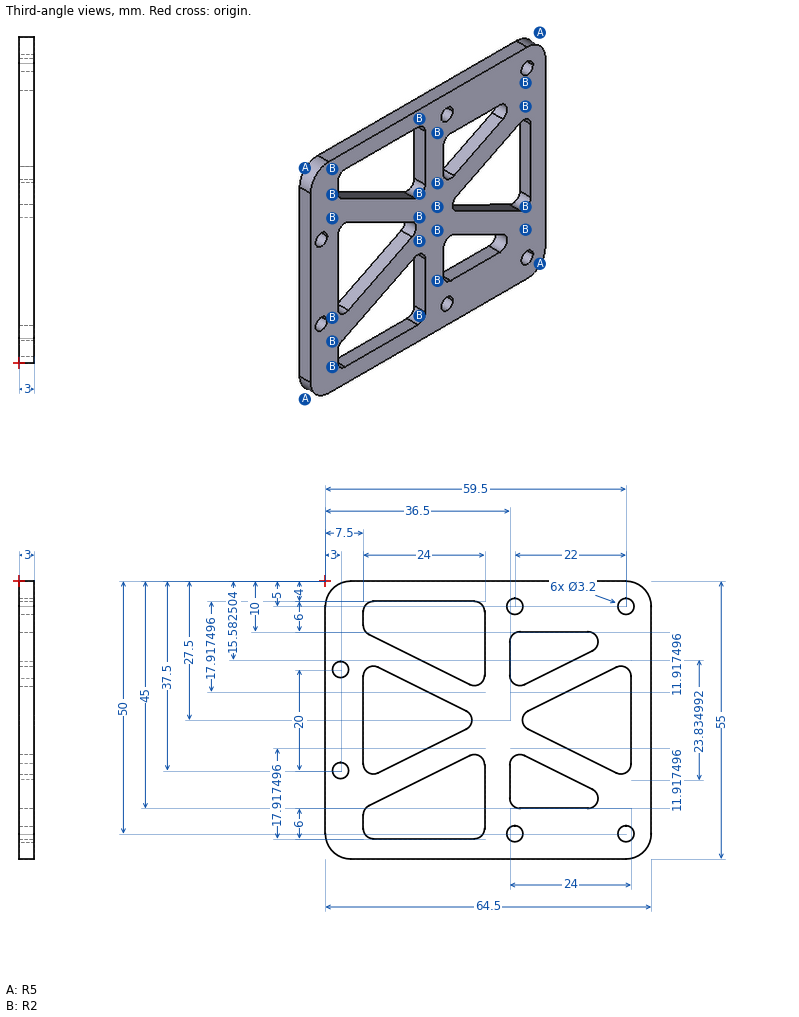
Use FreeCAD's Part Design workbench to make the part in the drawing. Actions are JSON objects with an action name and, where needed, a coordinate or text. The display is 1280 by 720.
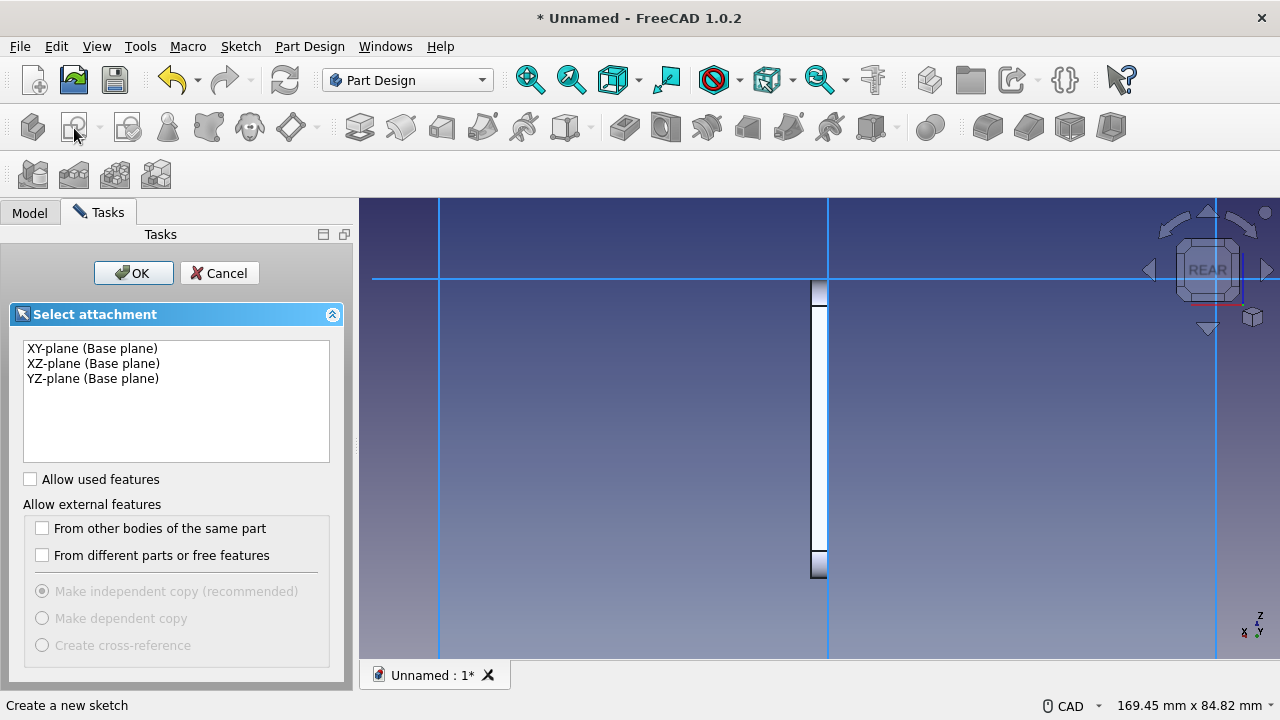
{"action": "left_click", "coordinate": [84, 378]}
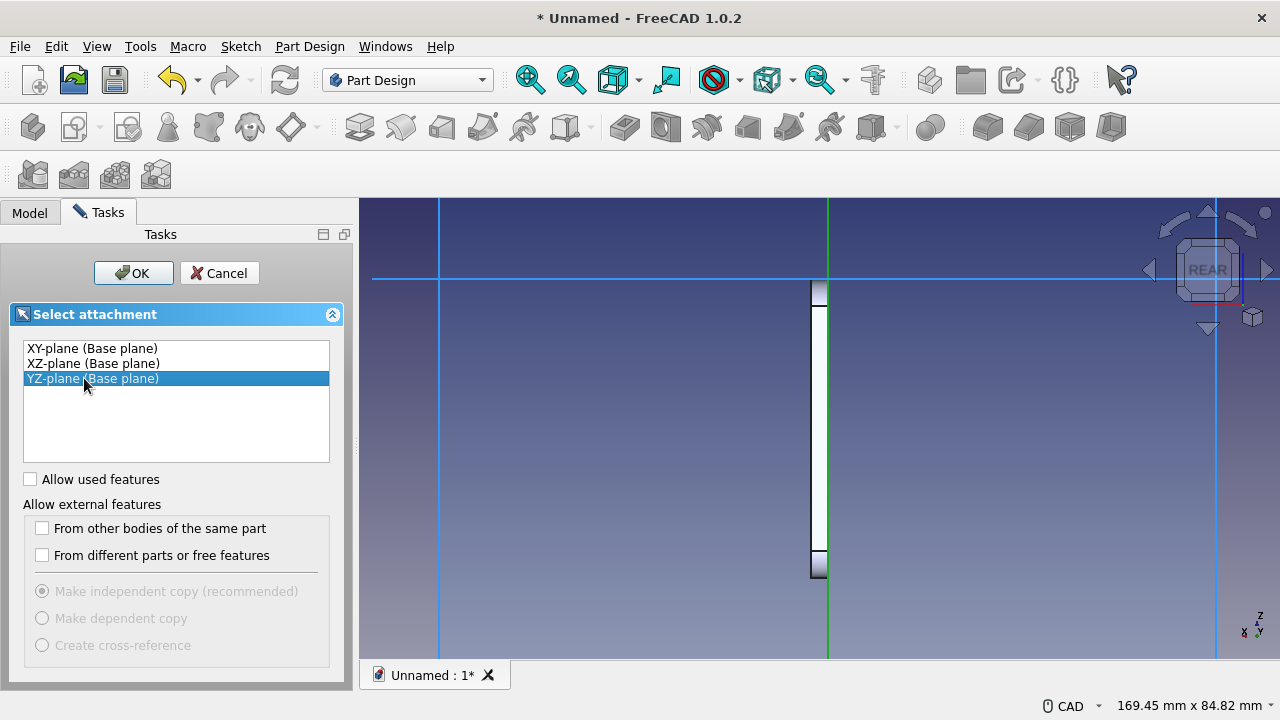
{"action": "left_click", "coordinate": [134, 273]}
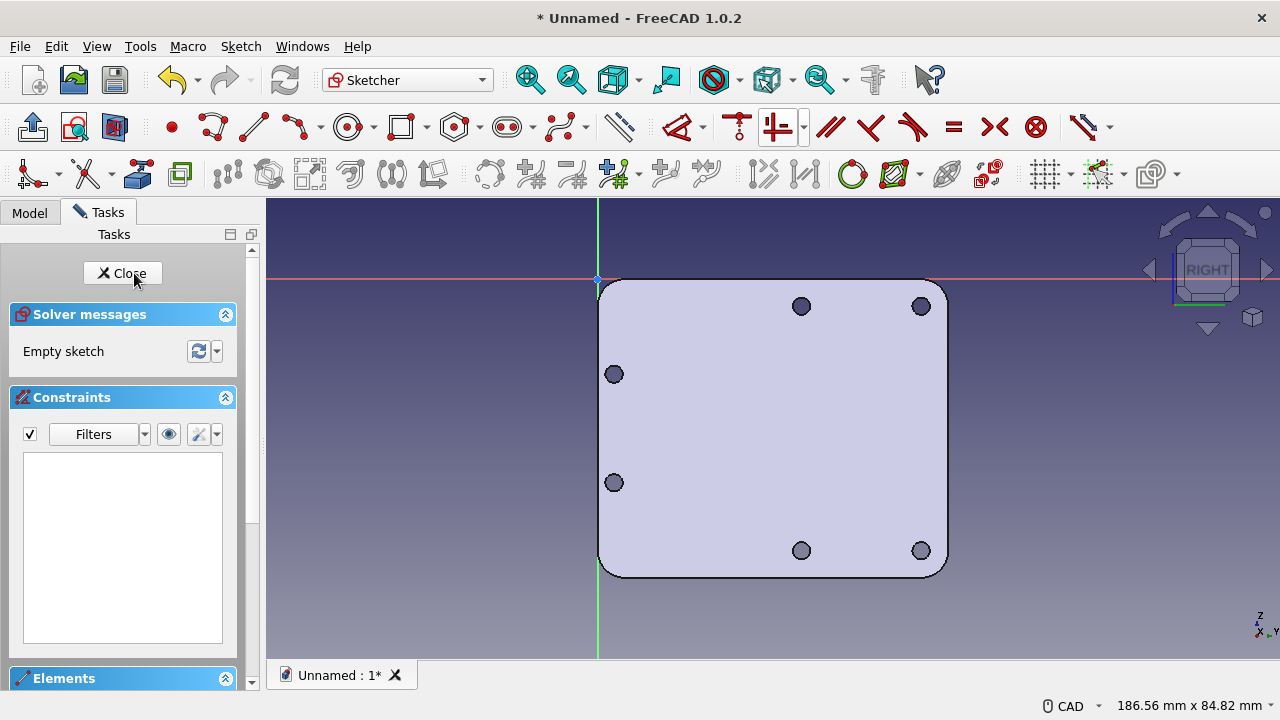
{"action": "key", "text": "q s"}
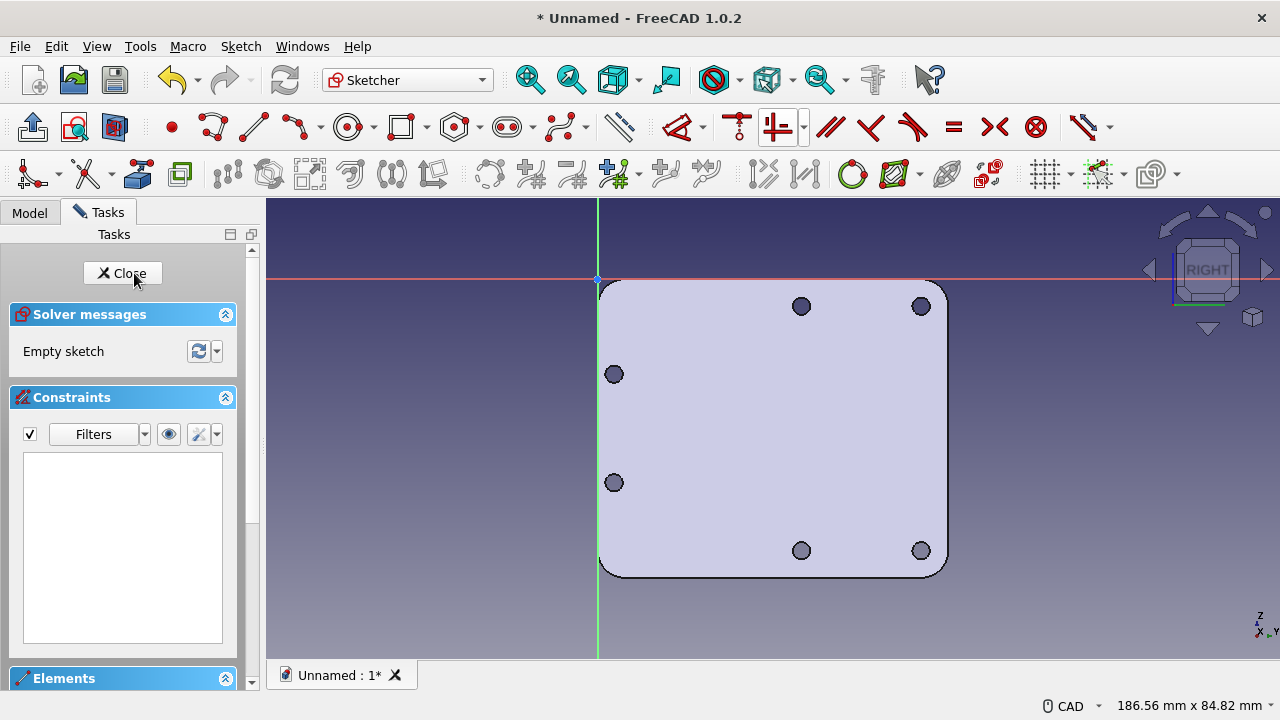
{"action": "key", "text": "g m"}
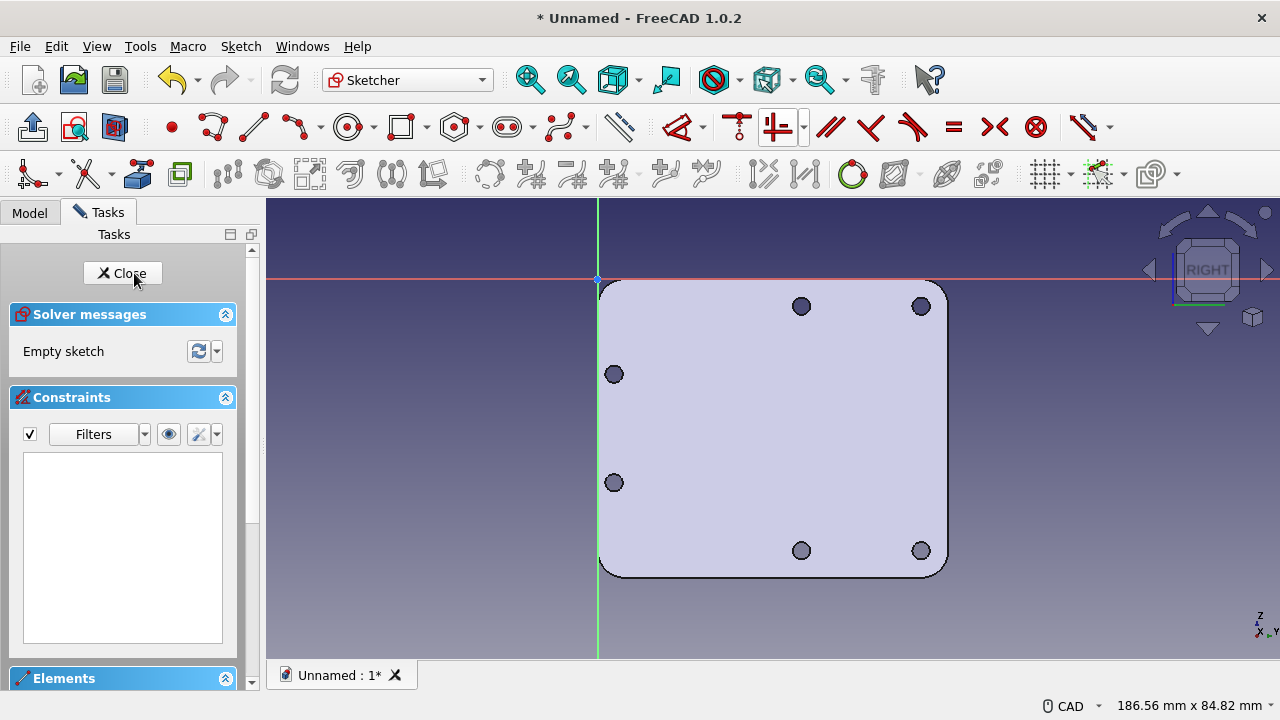
{"action": "left_click", "coordinate": [796, 428]}
{"action": "left_click", "coordinate": [927, 364]}
{"action": "left_click", "coordinate": [927, 493]}
{"action": "left_click", "coordinate": [796, 429]}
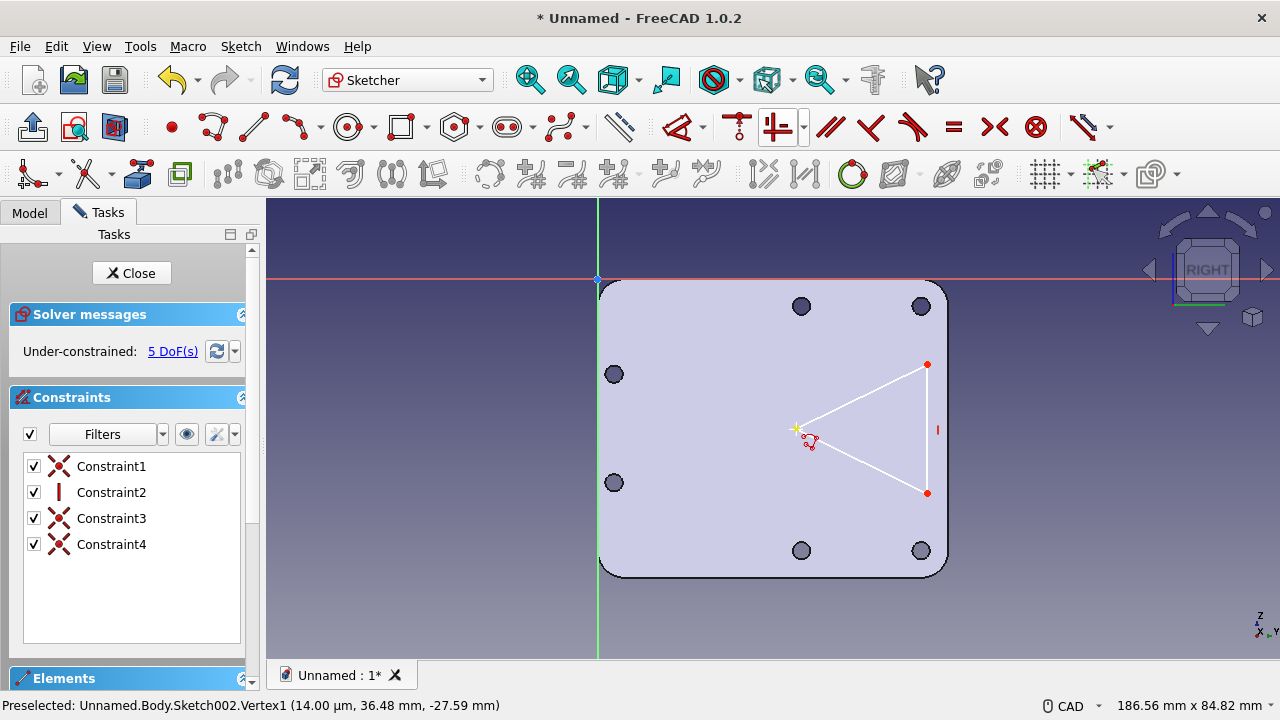
{"action": "left_click", "coordinate": [796, 459]}
{"action": "left_click", "coordinate": [927, 524]}
{"action": "left_click", "coordinate": [796, 524]}
{"action": "left_click", "coordinate": [796, 460]}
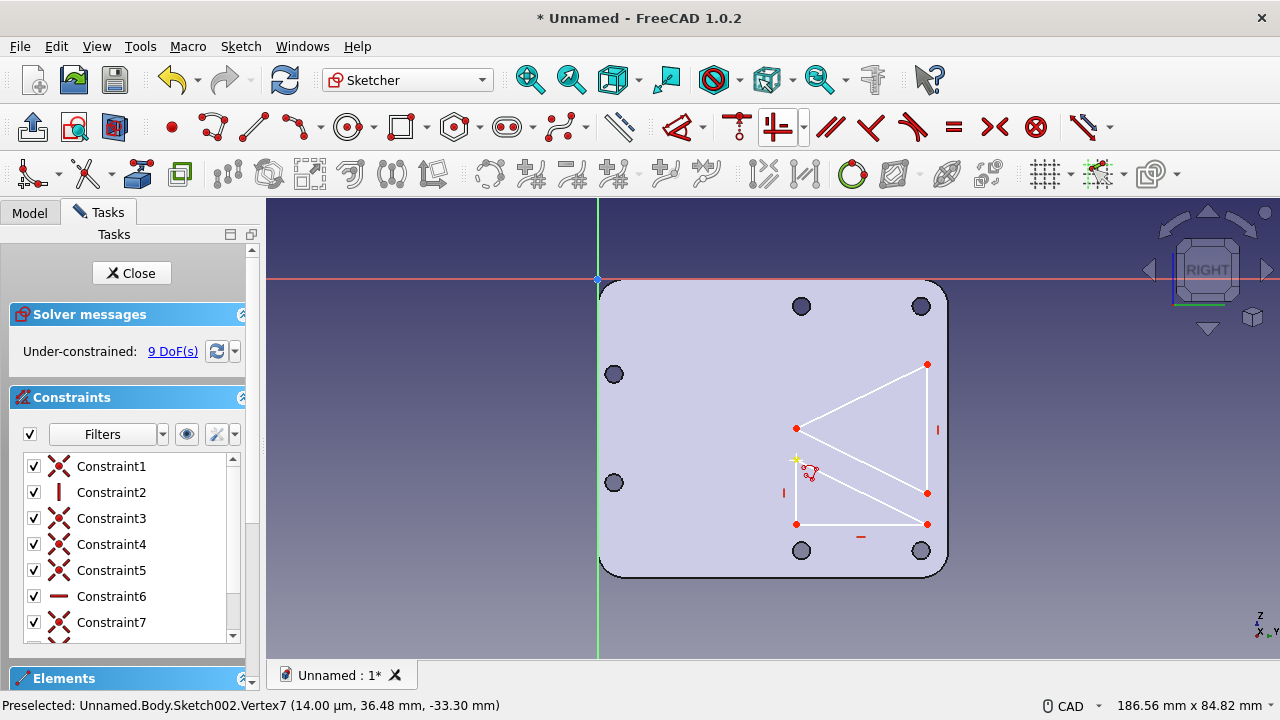
{"action": "left_click", "coordinate": [796, 333]}
{"action": "left_click", "coordinate": [927, 333]}
{"action": "left_click", "coordinate": [796, 398]}
{"action": "left_click", "coordinate": [796, 334]}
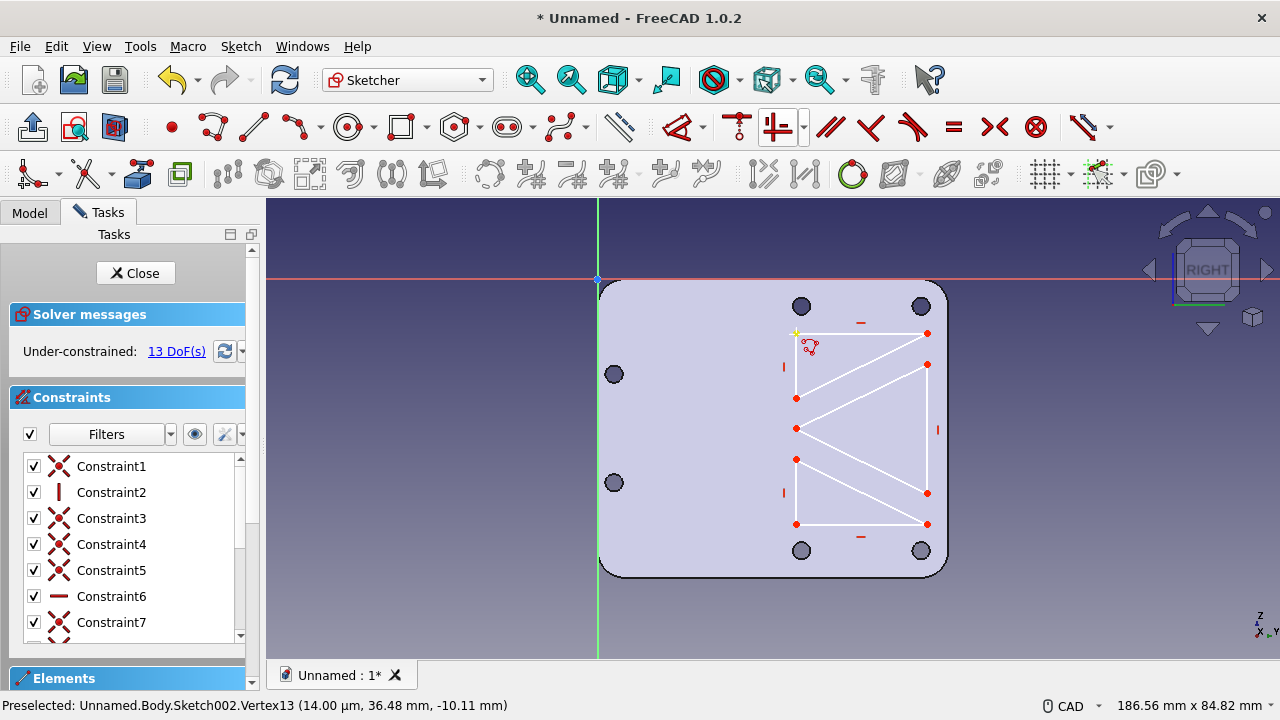
{"action": "left_click", "coordinate": [638, 301]}
{"action": "left_click", "coordinate": [769, 301]}
{"action": "left_click", "coordinate": [769, 398]}
{"action": "left_click", "coordinate": [638, 333]}
{"action": "left_click", "coordinate": [638, 302]}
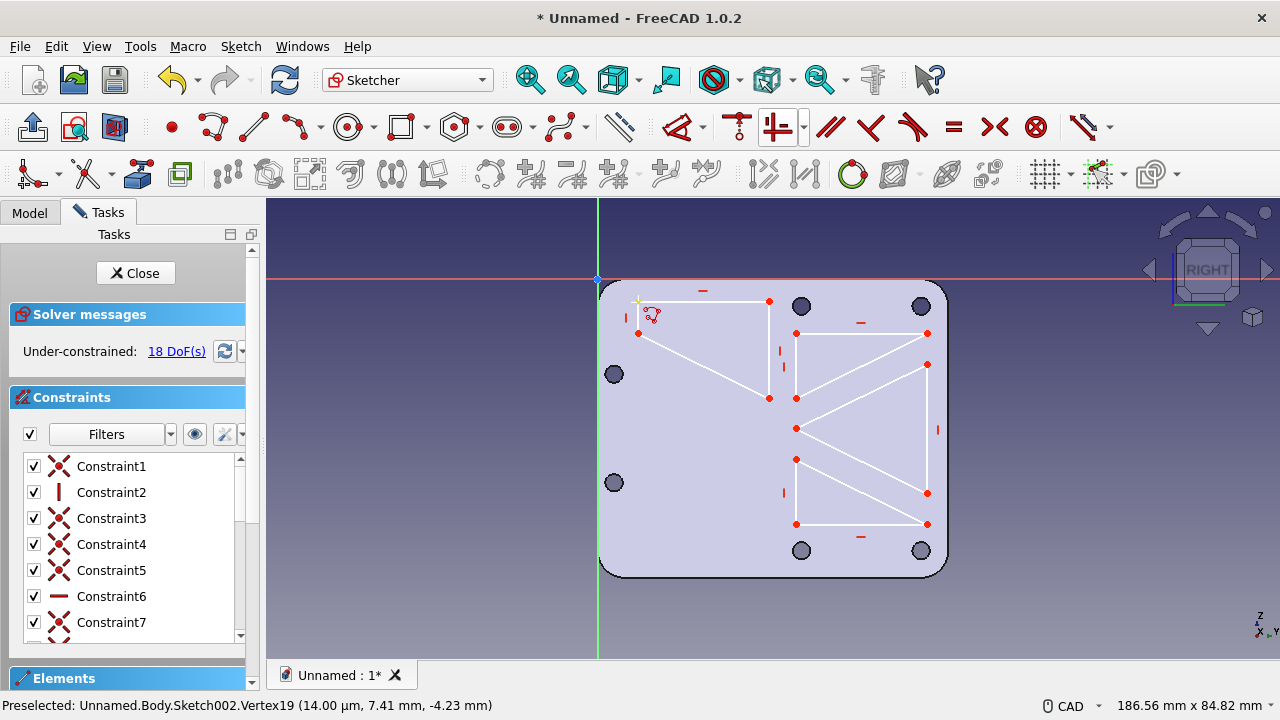
{"action": "left_click", "coordinate": [638, 364]}
{"action": "left_click", "coordinate": [769, 428]}
{"action": "left_click", "coordinate": [638, 493]}
{"action": "left_click", "coordinate": [638, 365]}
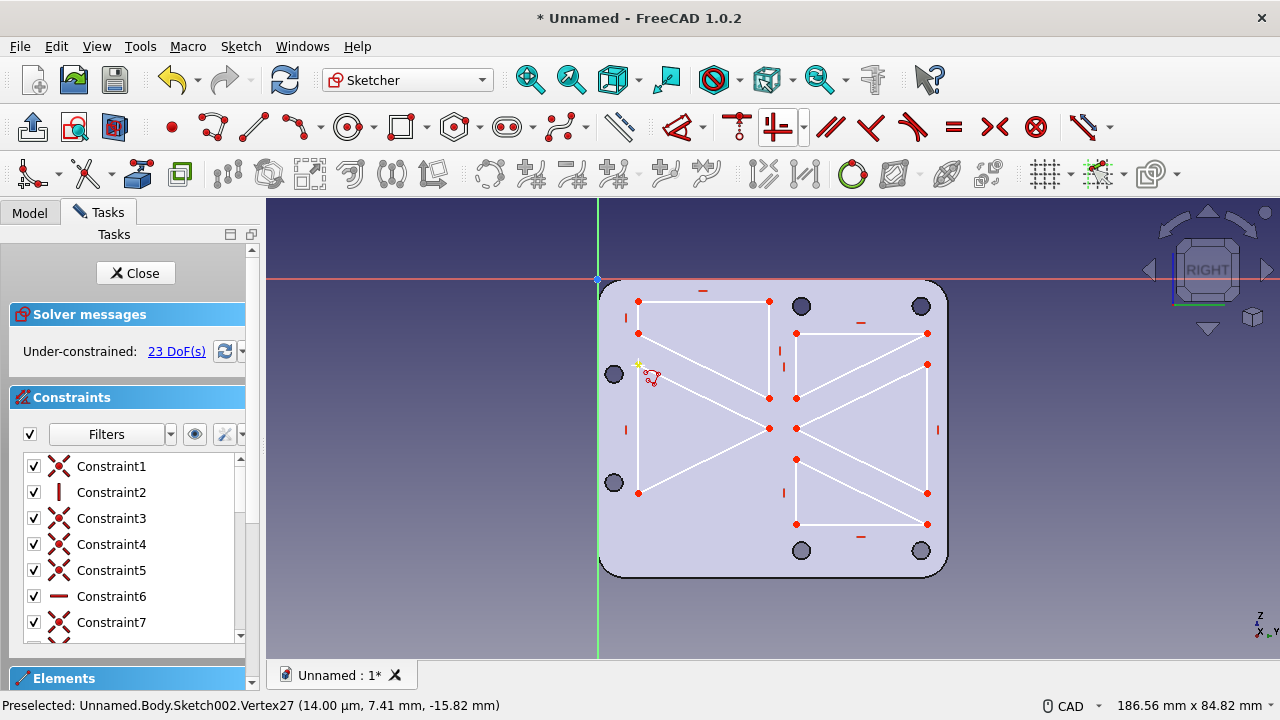
{"action": "left_click", "coordinate": [638, 524]}
{"action": "left_click", "coordinate": [769, 459]}
{"action": "left_click", "coordinate": [769, 556]}
{"action": "left_click", "coordinate": [638, 556]}
{"action": "left_click", "coordinate": [638, 525]}
{"action": "key", "text": "Escape"}
{"action": "key", "text": "Escape"}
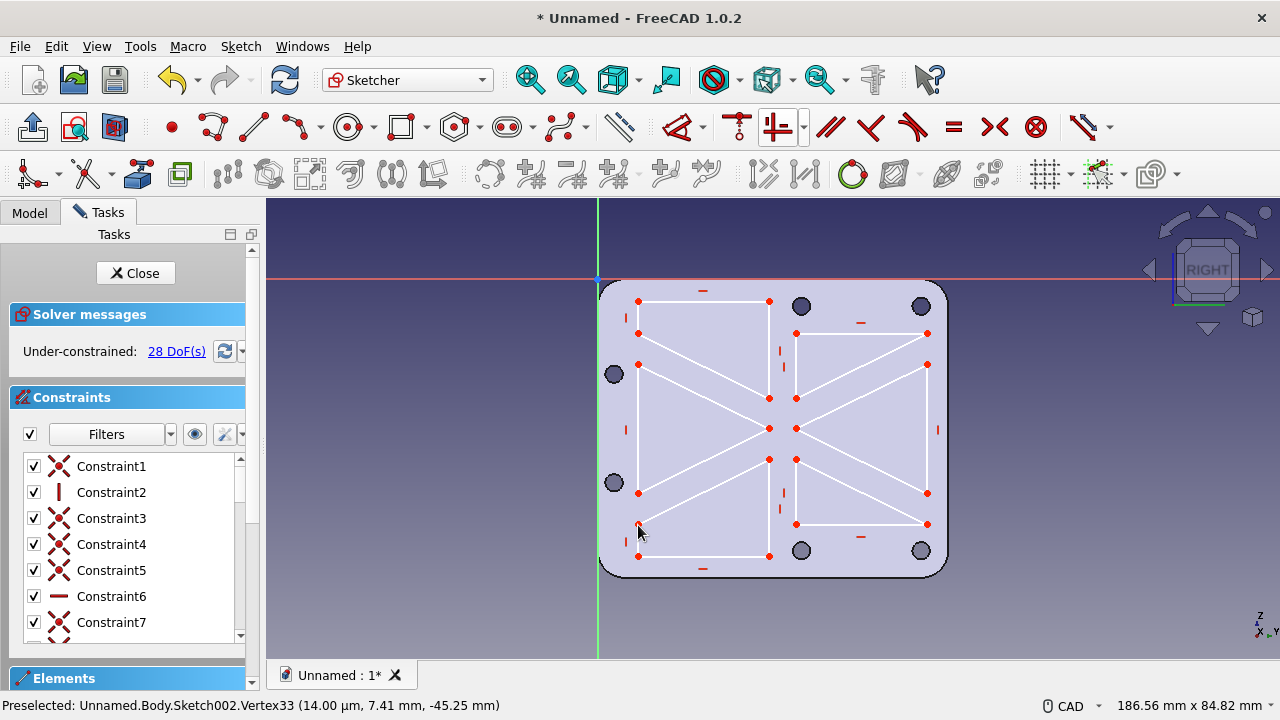
{"action": "left_click", "coordinate": [676, 128]}